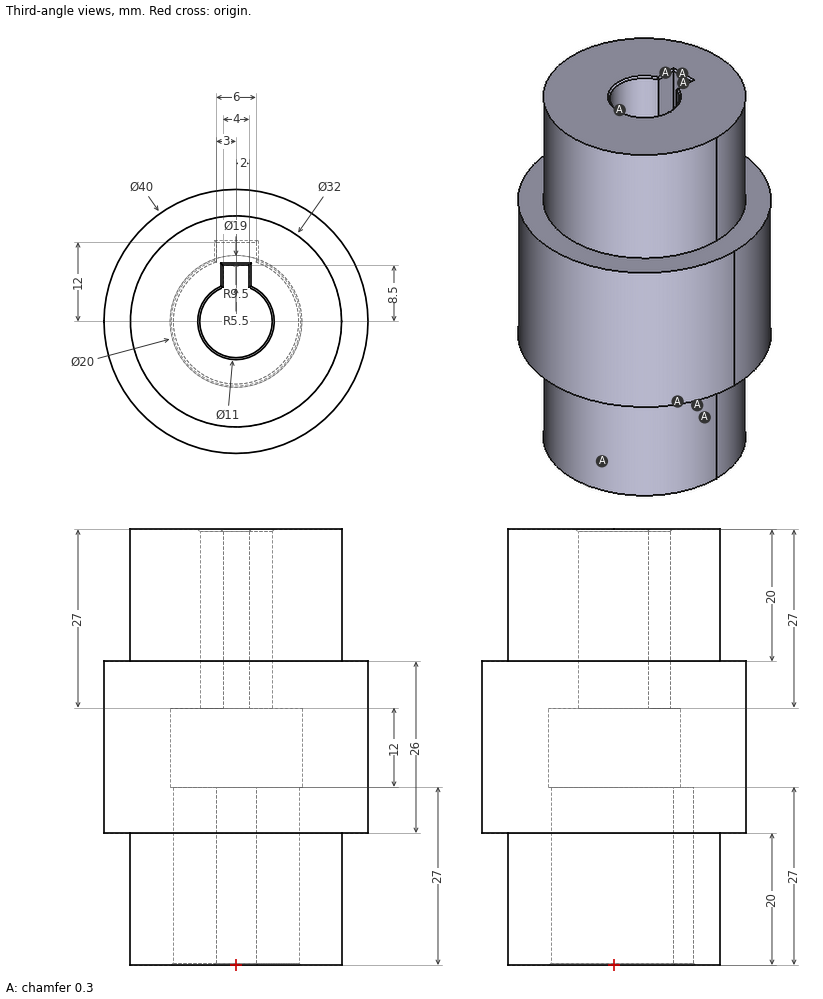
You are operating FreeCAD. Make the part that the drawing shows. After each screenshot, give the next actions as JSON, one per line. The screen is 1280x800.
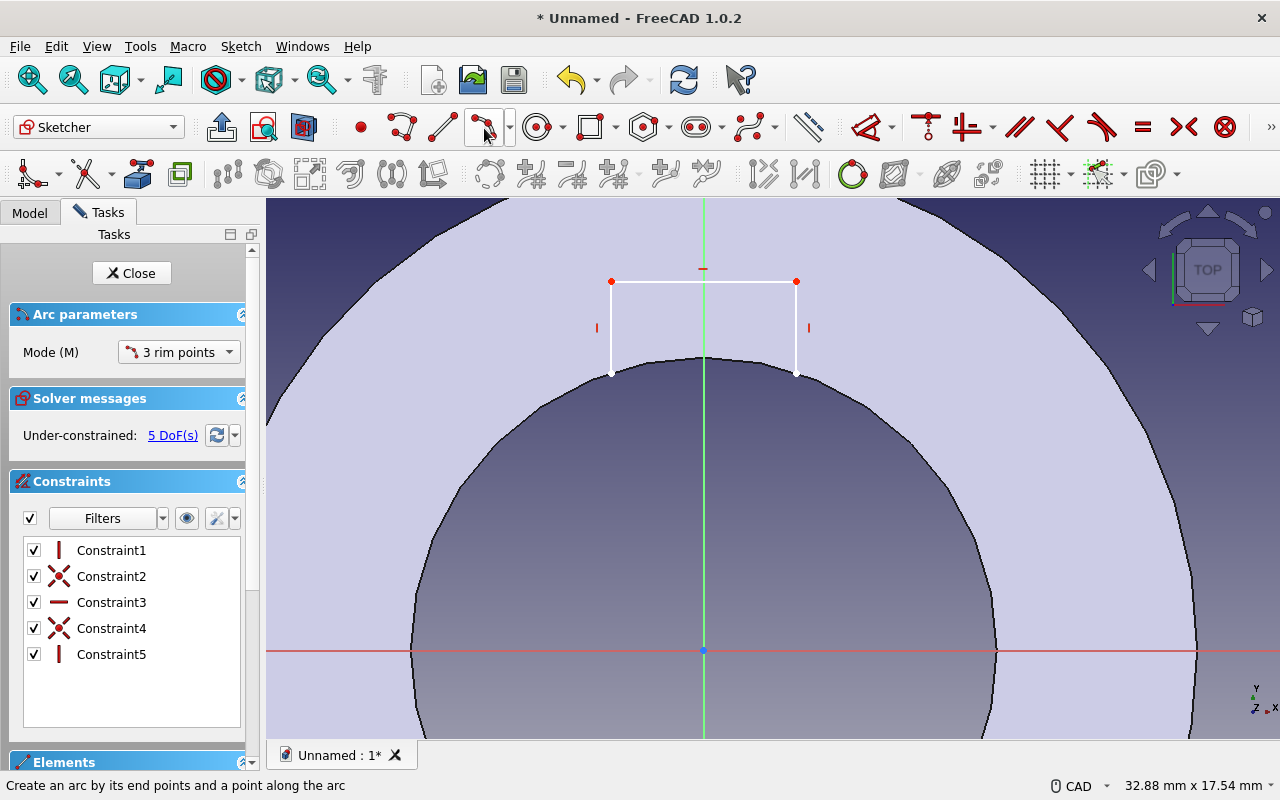
{"action": "left_click", "coordinate": [796, 374]}
{"action": "left_click", "coordinate": [611, 374]}
{"action": "left_click", "coordinate": [723, 358]}
{"action": "key", "text": "Escape"}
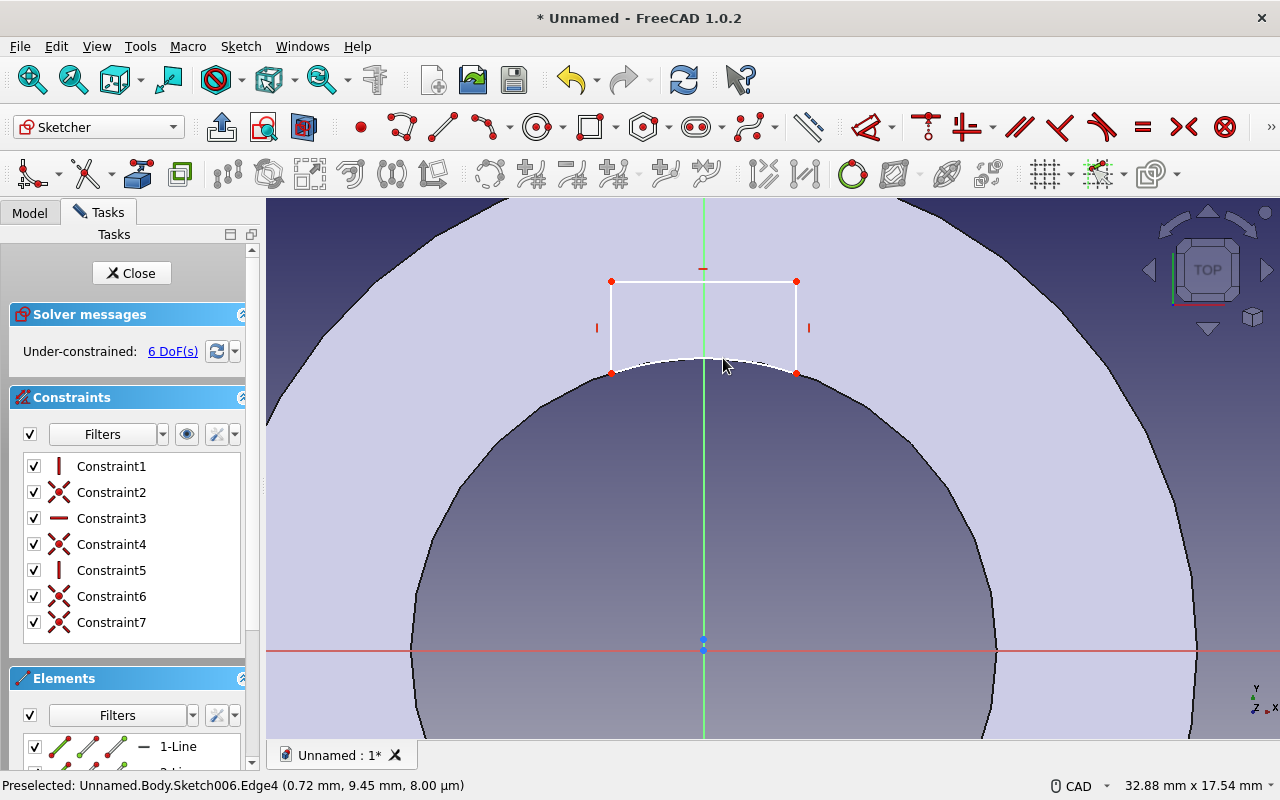
{"action": "left_click_drag", "start_coordinate": [694, 629], "coordinate": [714, 661]}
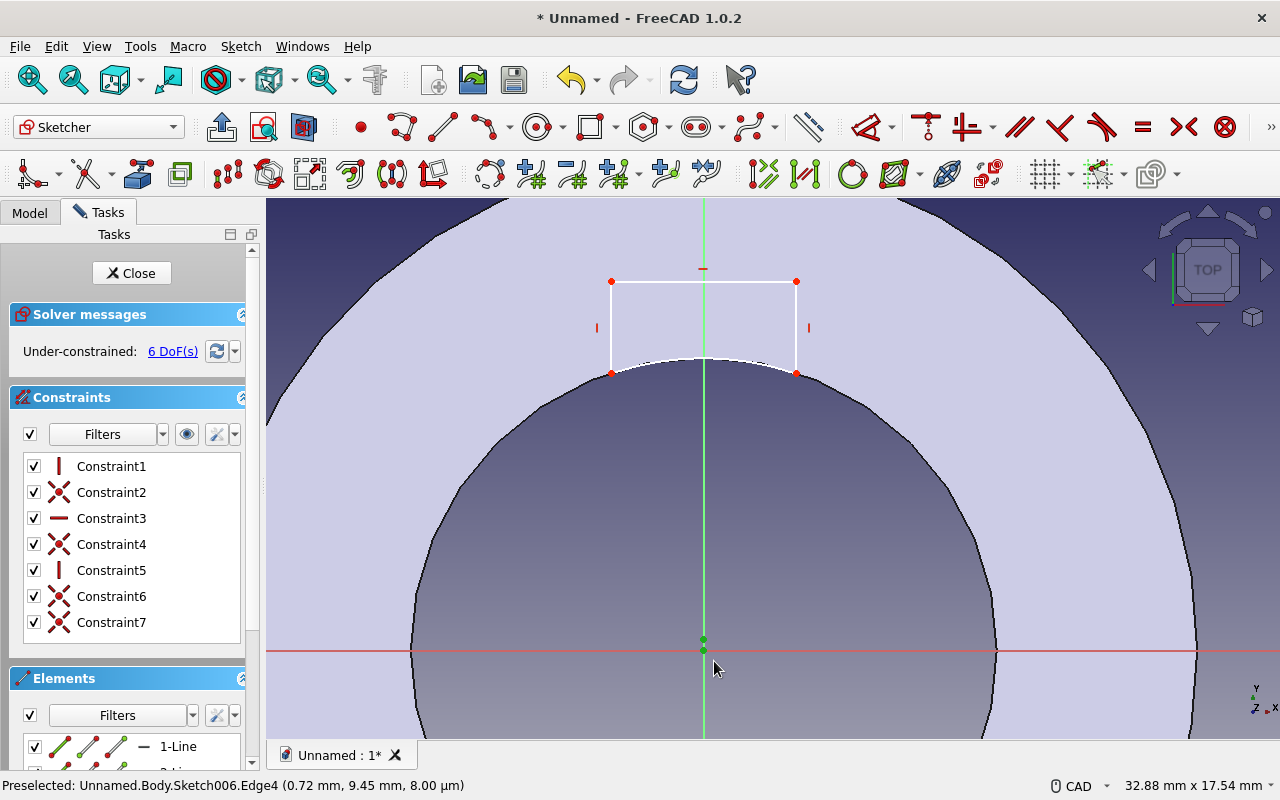
{"action": "left_click", "coordinate": [926, 128]}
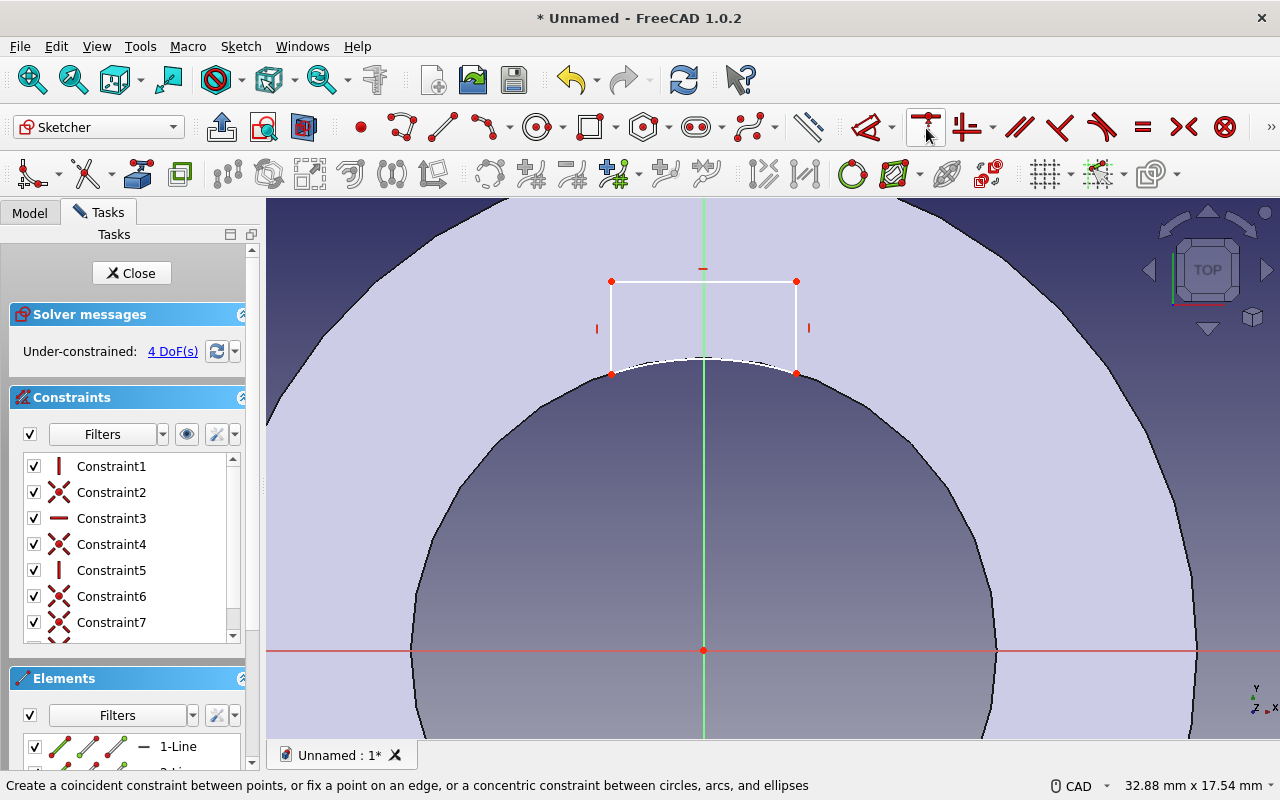
{"action": "left_click", "coordinate": [866, 128]}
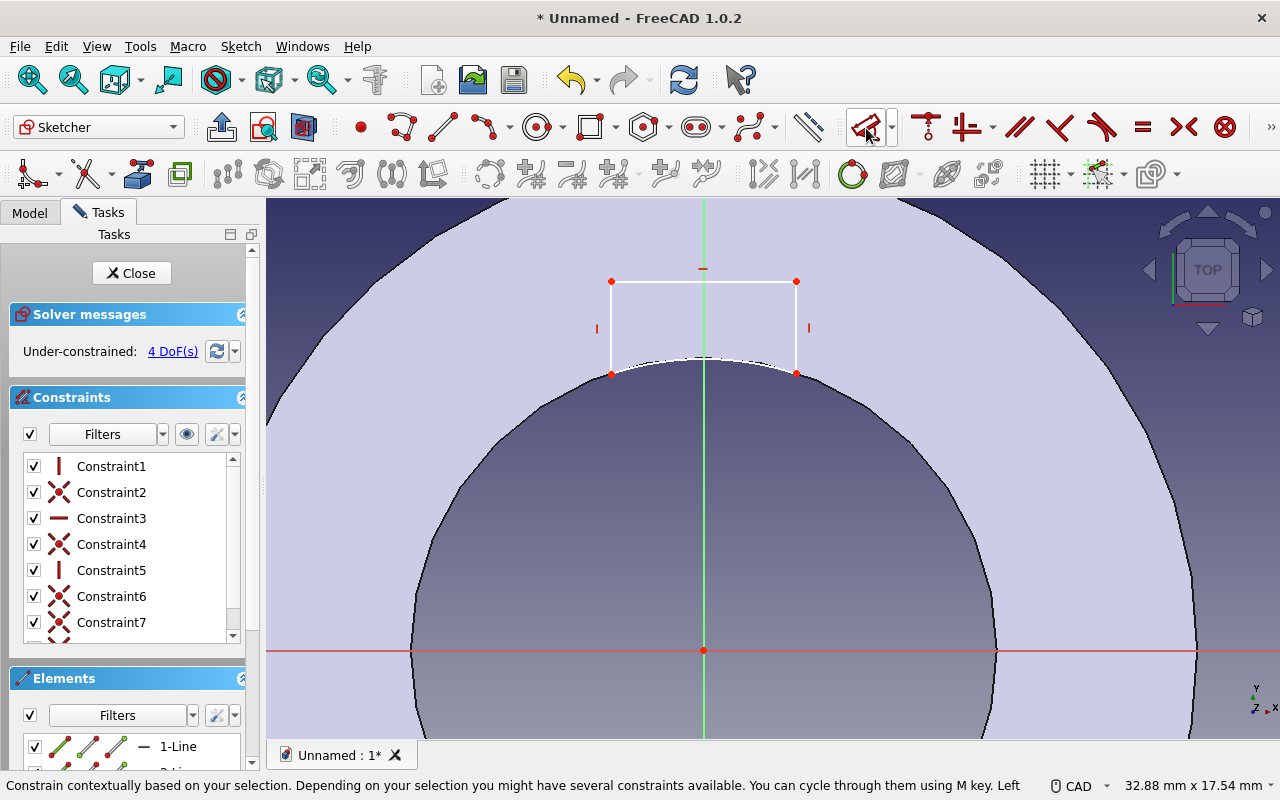
{"action": "left_click", "coordinate": [741, 361]}
{"action": "left_click", "coordinate": [745, 329]}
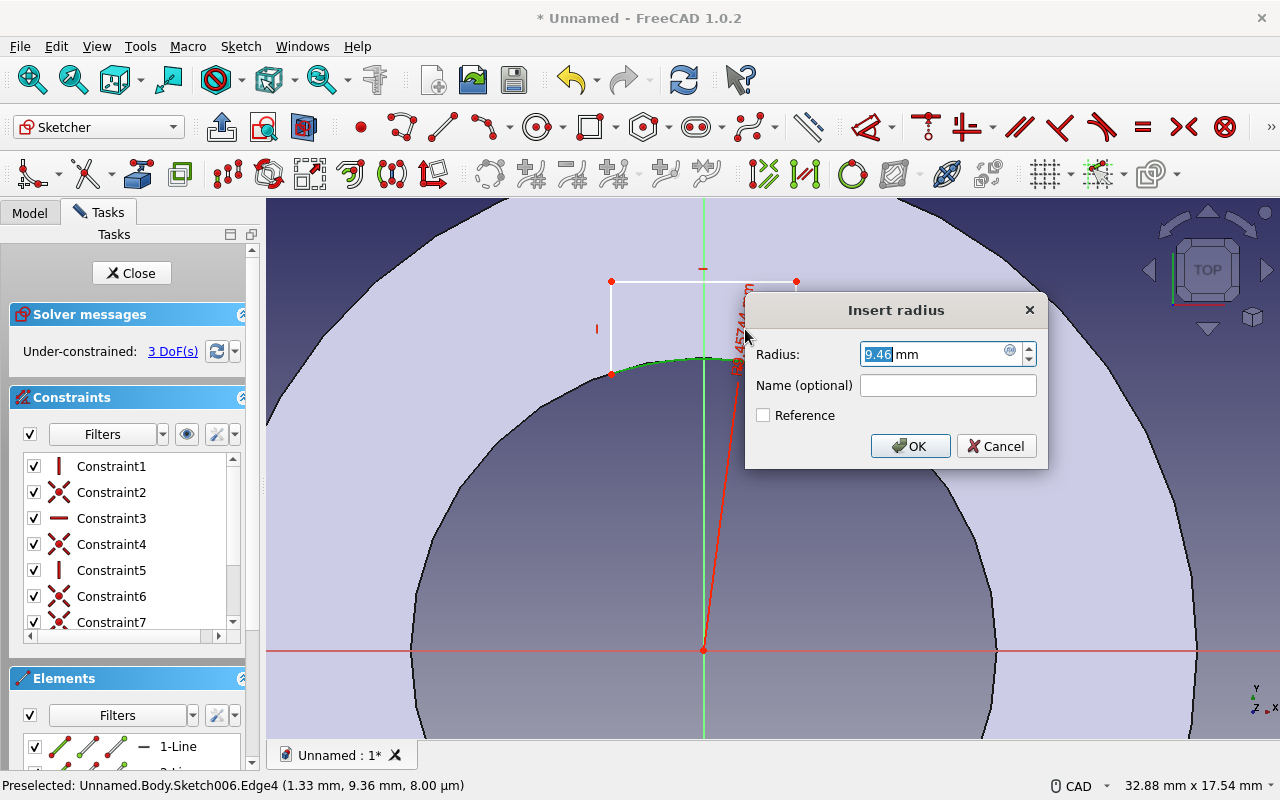
{"action": "type", "text": "9.5"}
{"action": "key", "text": "Return"}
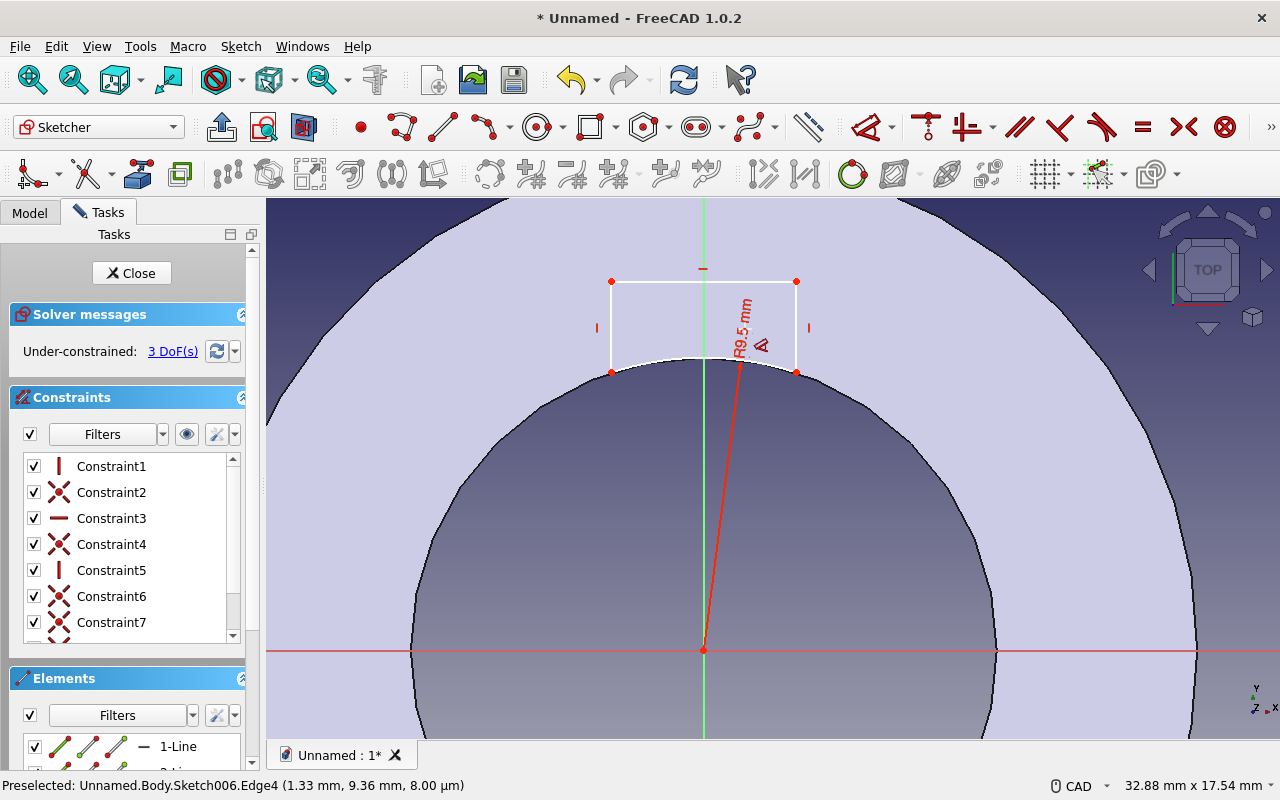
{"action": "left_click", "coordinate": [667, 282]}
{"action": "left_click", "coordinate": [661, 248]}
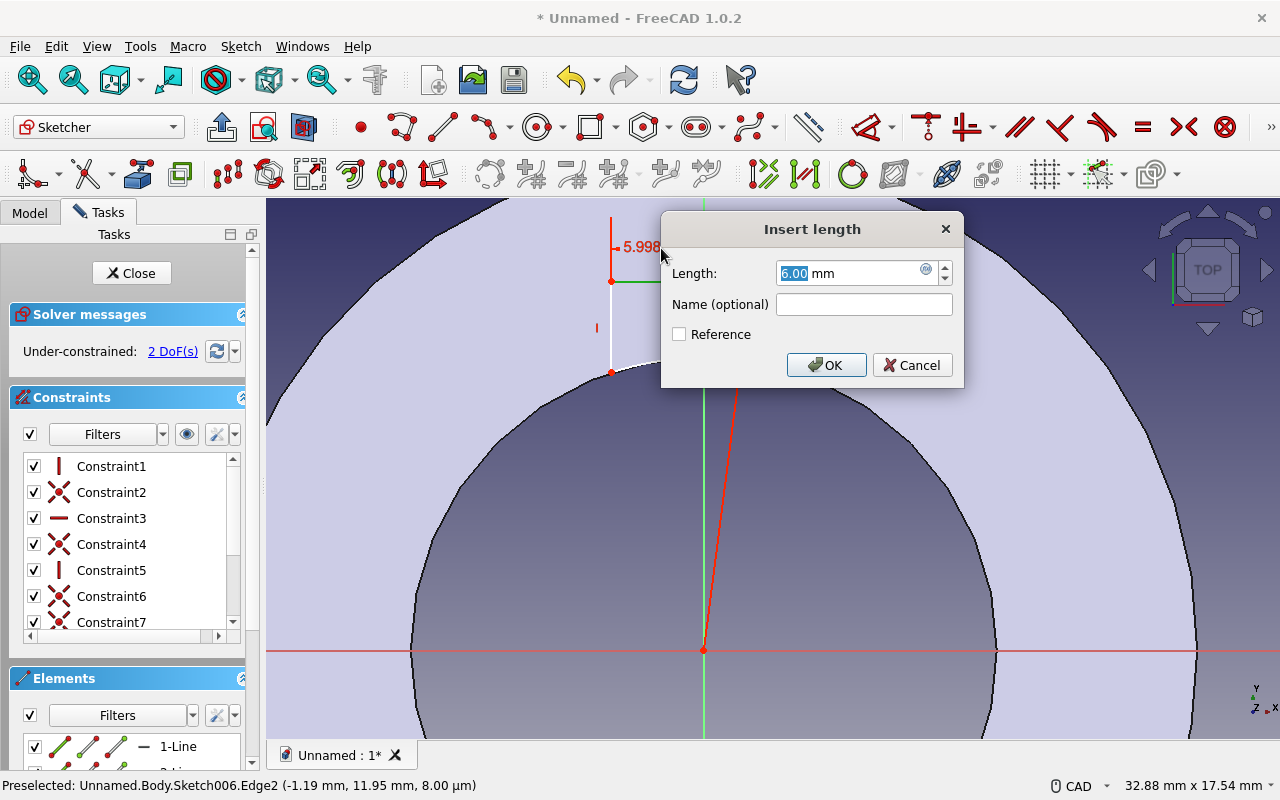
{"action": "type", "text": "6"}
{"action": "key", "text": "Return"}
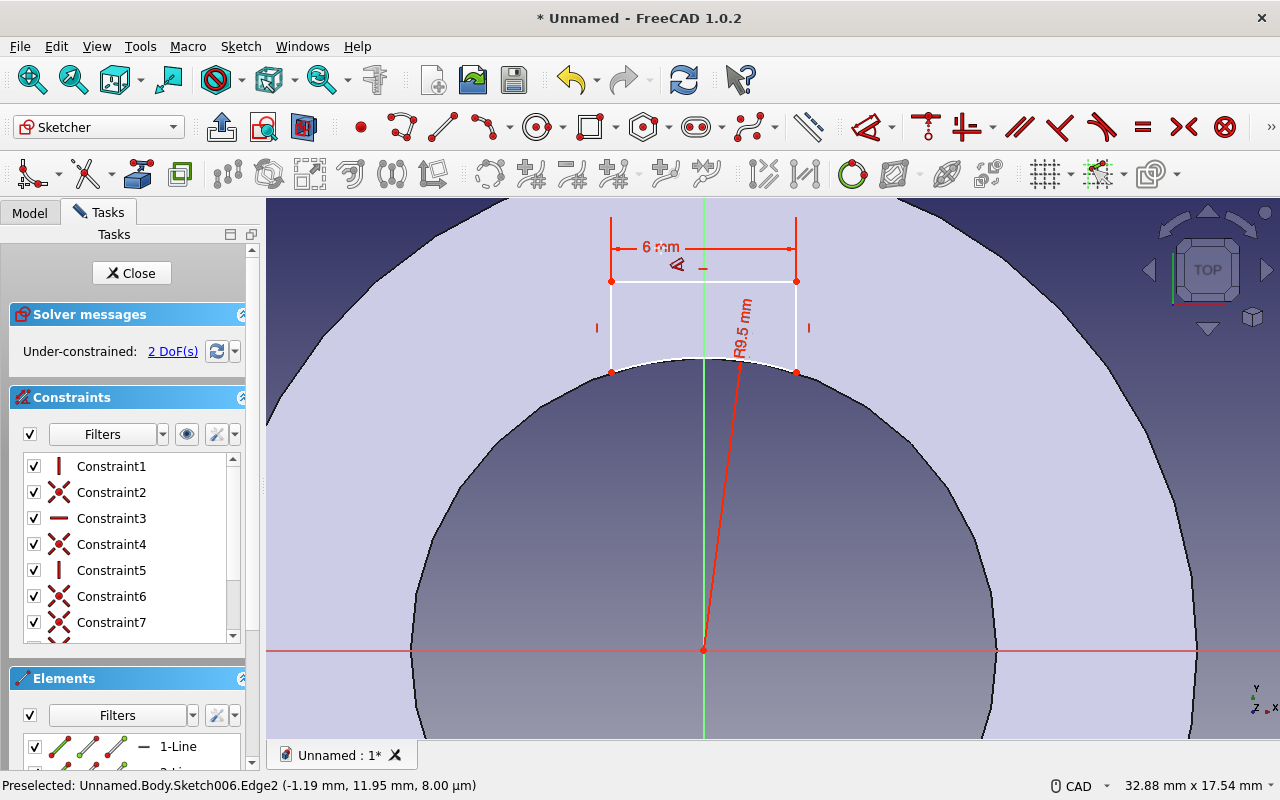
{"action": "left_click", "coordinate": [611, 373]}
{"action": "left_click", "coordinate": [657, 685]}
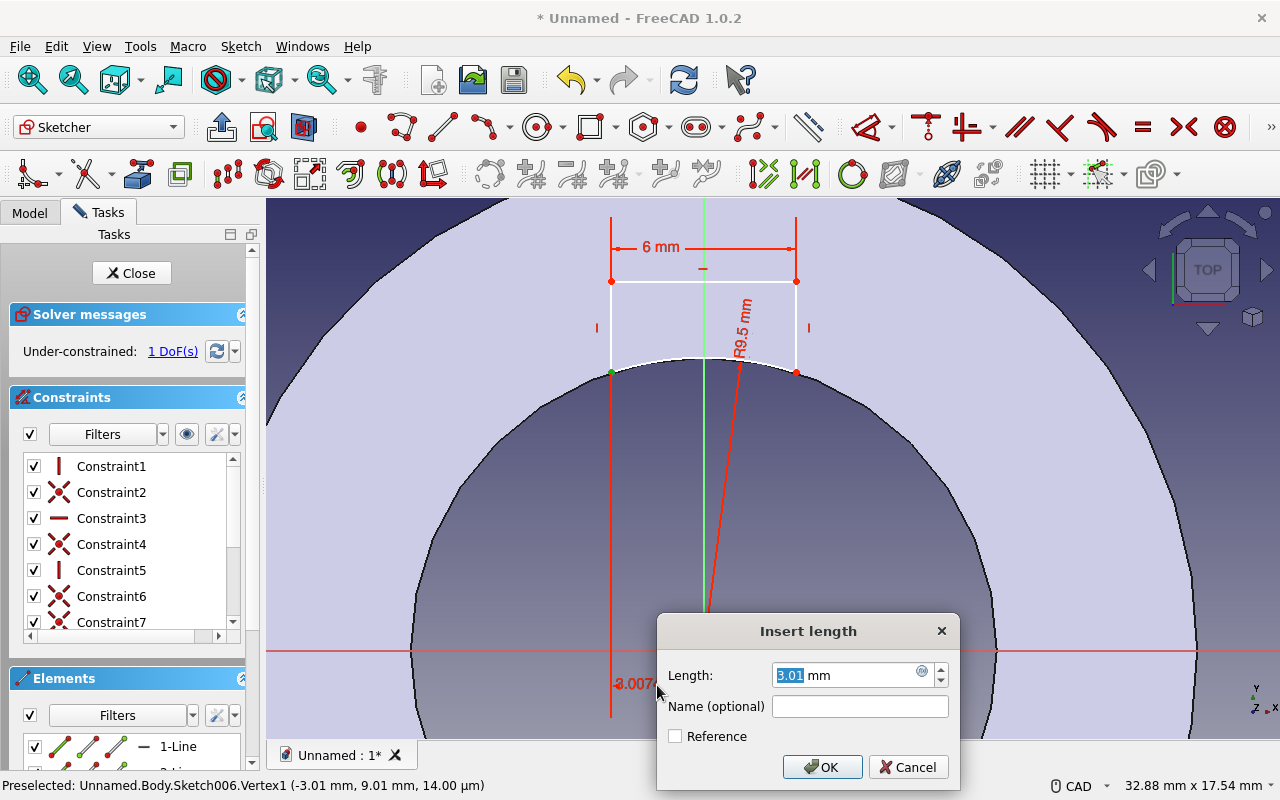
{"action": "type", "text": "3"}
{"action": "key", "text": "Return"}